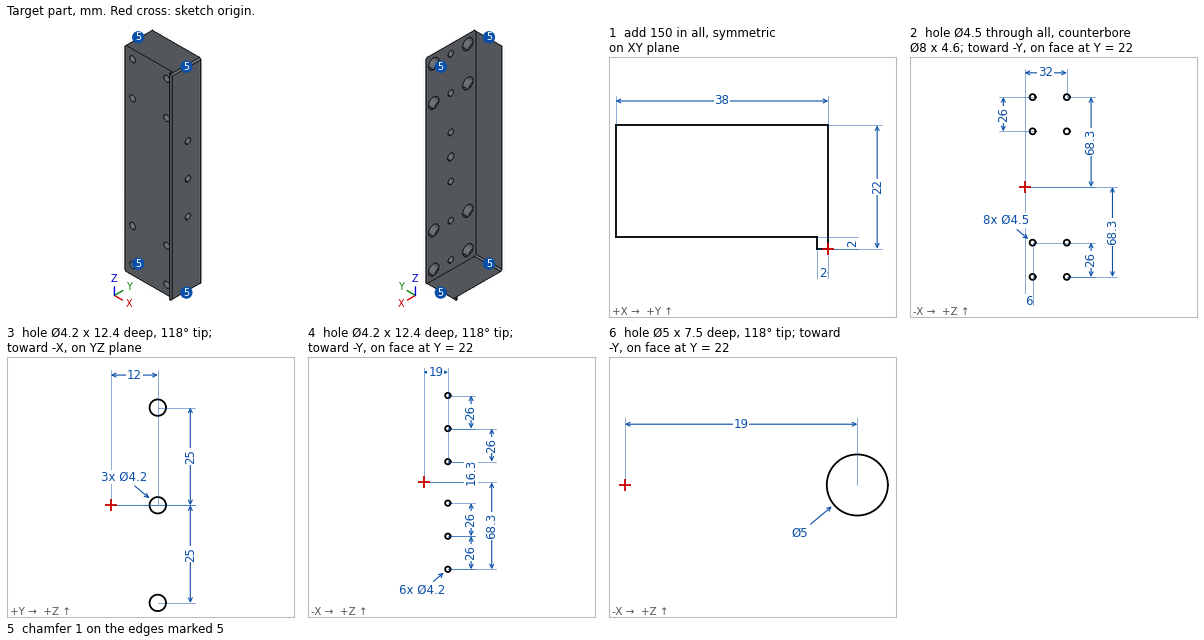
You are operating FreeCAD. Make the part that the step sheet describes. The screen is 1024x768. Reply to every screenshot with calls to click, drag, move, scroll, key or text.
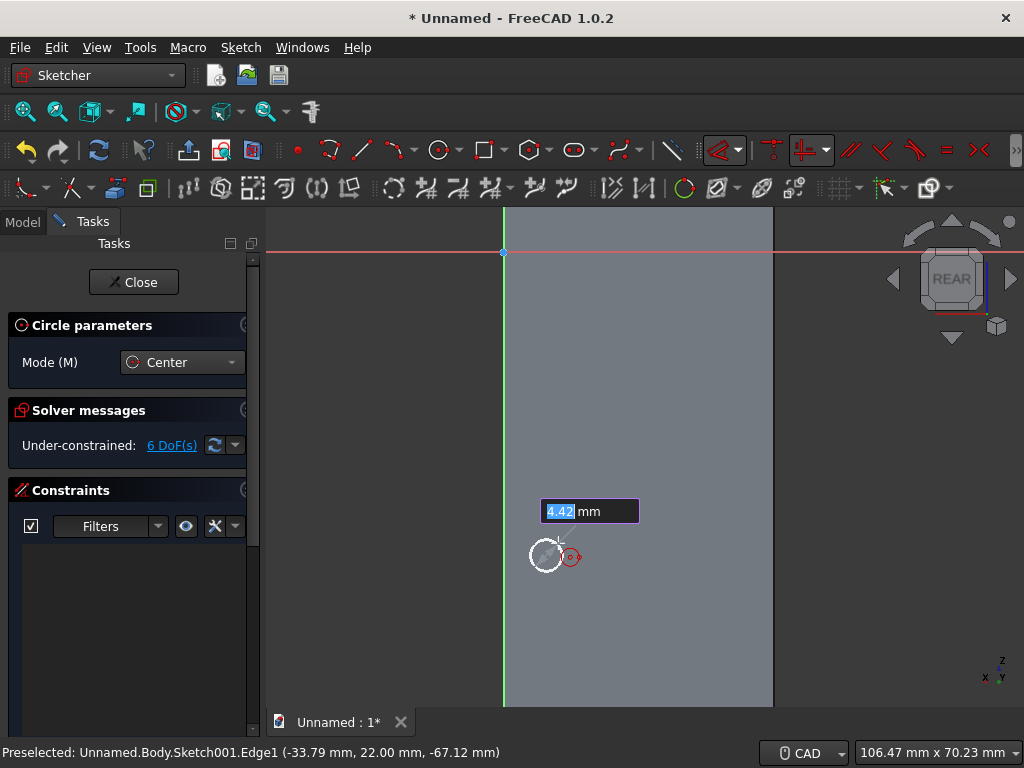
click(558, 542)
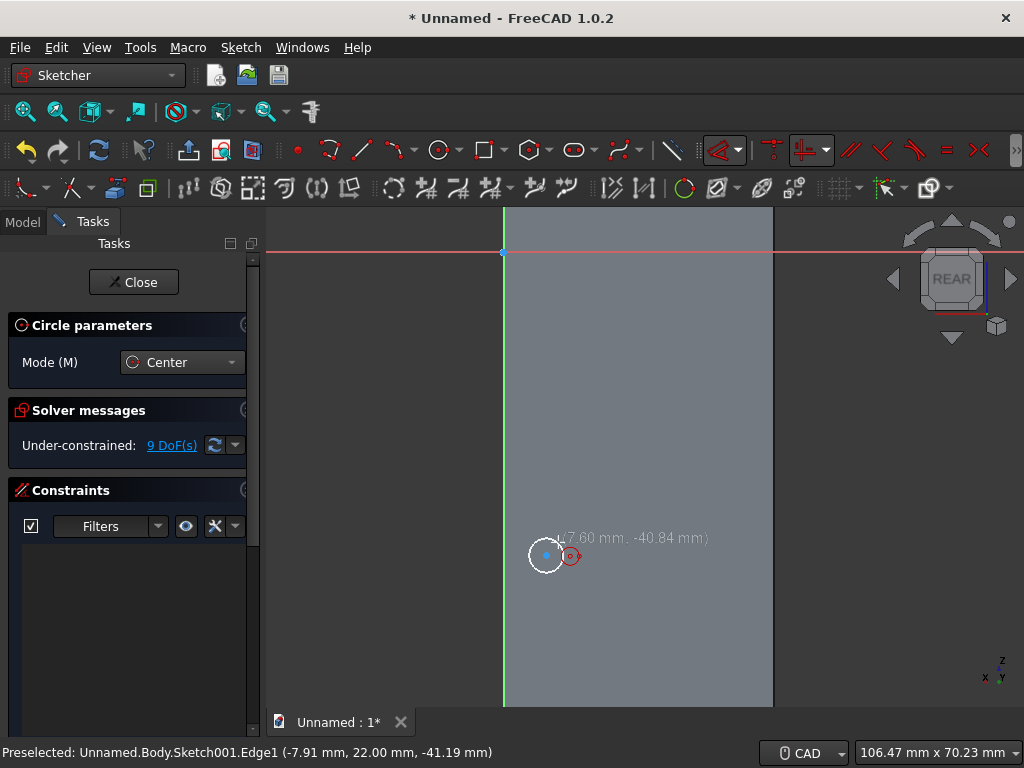
scroll(732, 553, up, 2)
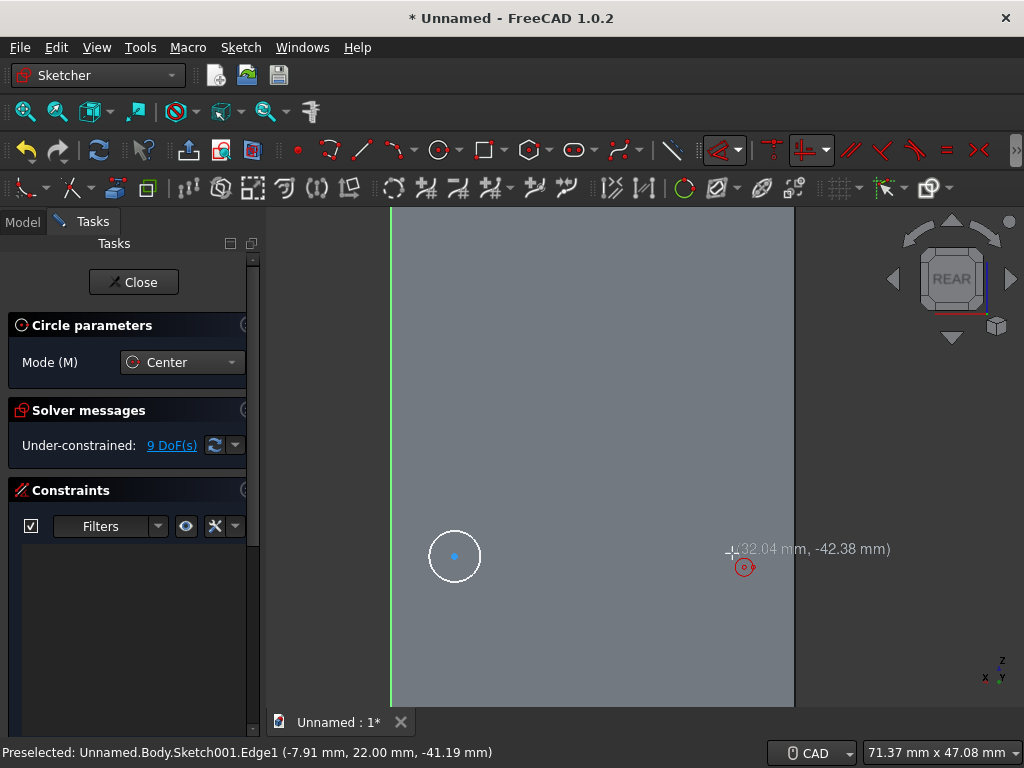
scroll(577, 546, down, 8)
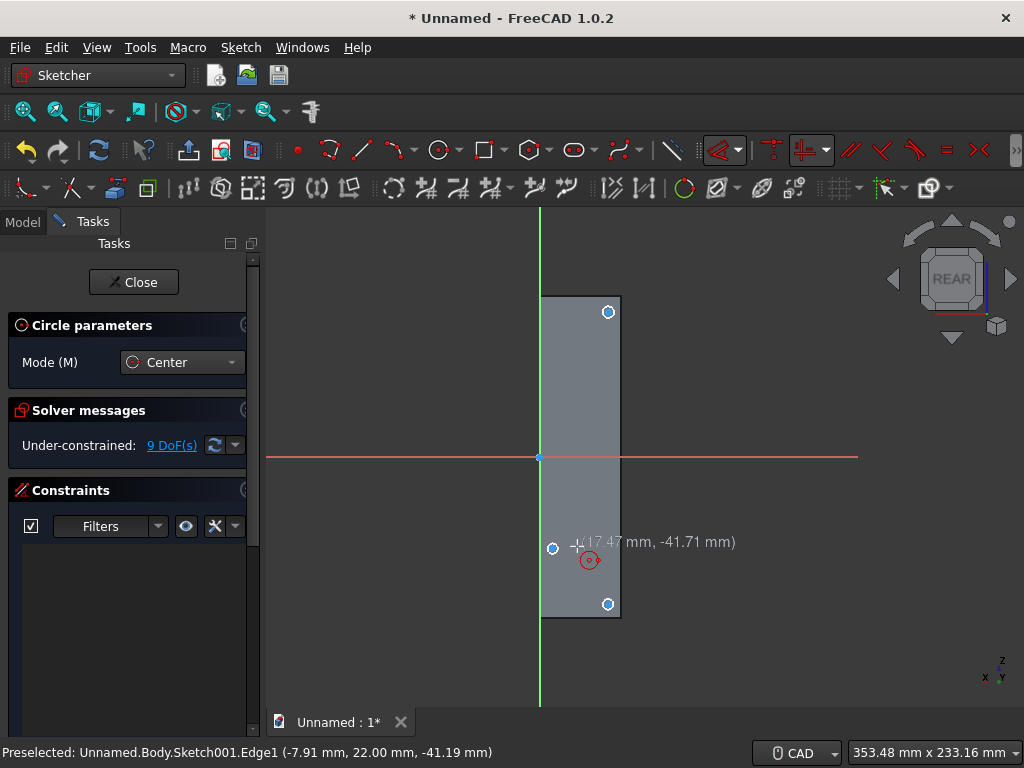
click(608, 548)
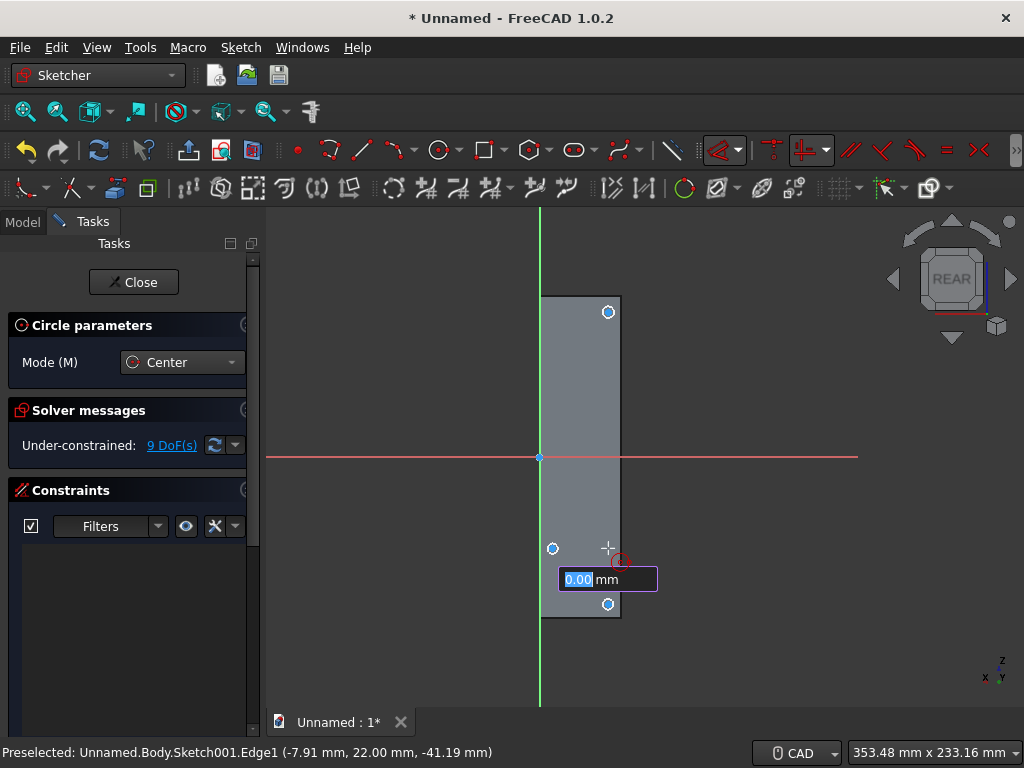
scroll(612, 545, up, 6)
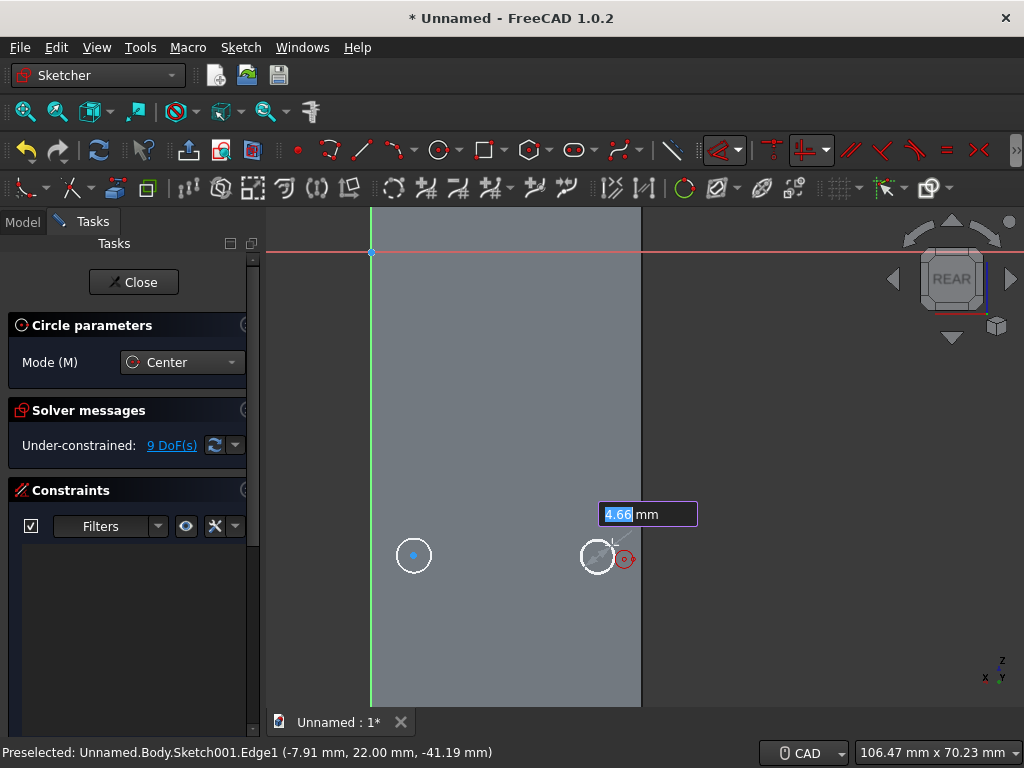
click(611, 542)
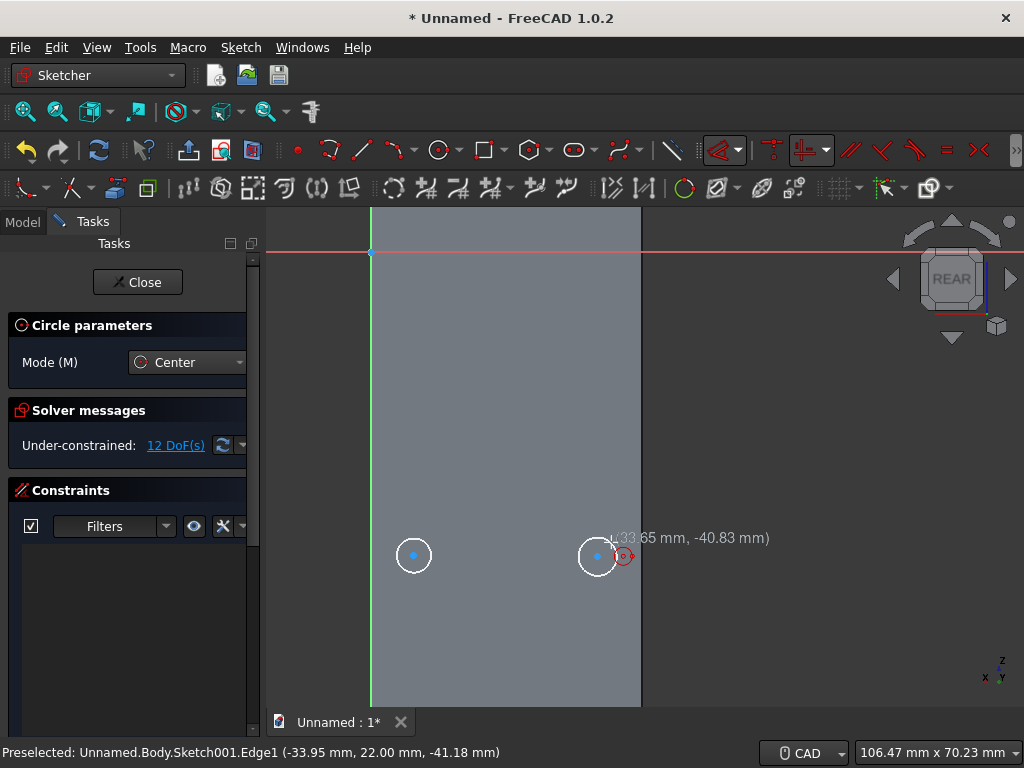
scroll(612, 545, down, 6)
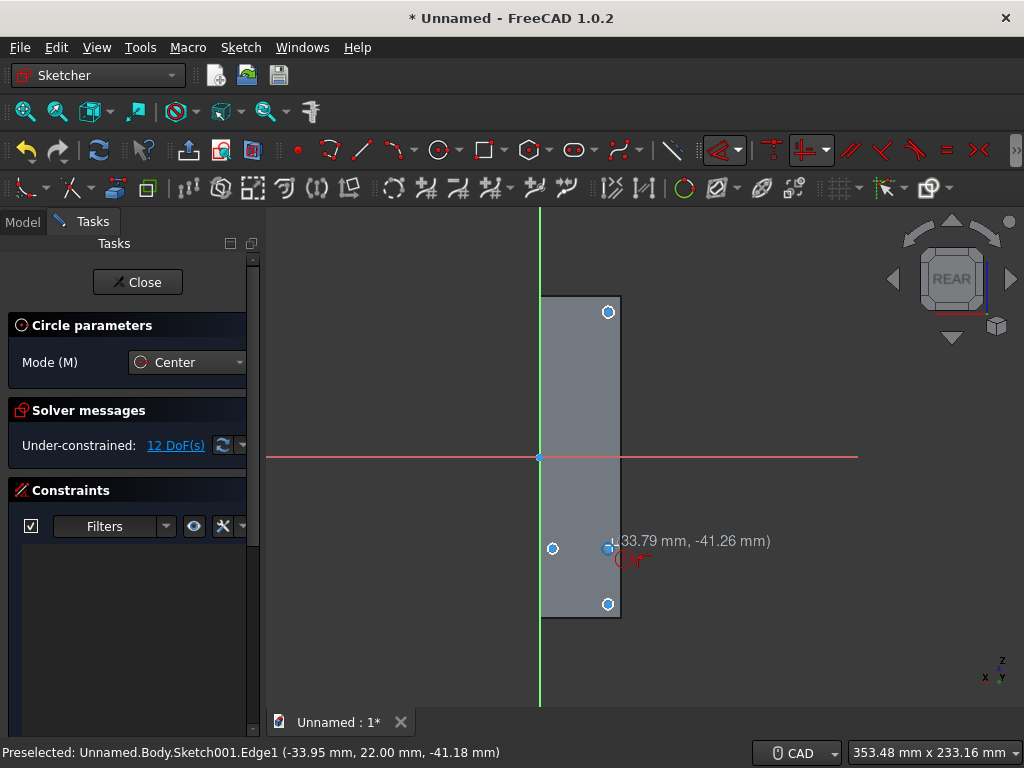
scroll(553, 604, up, 8)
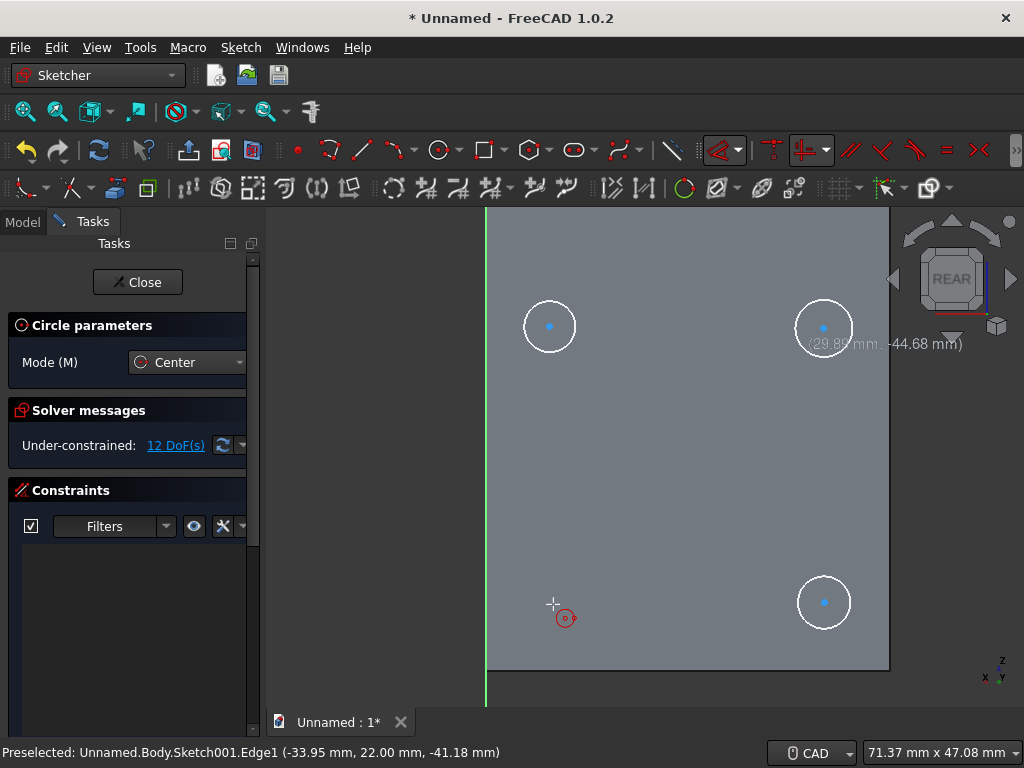
scroll(553, 604, down, 8)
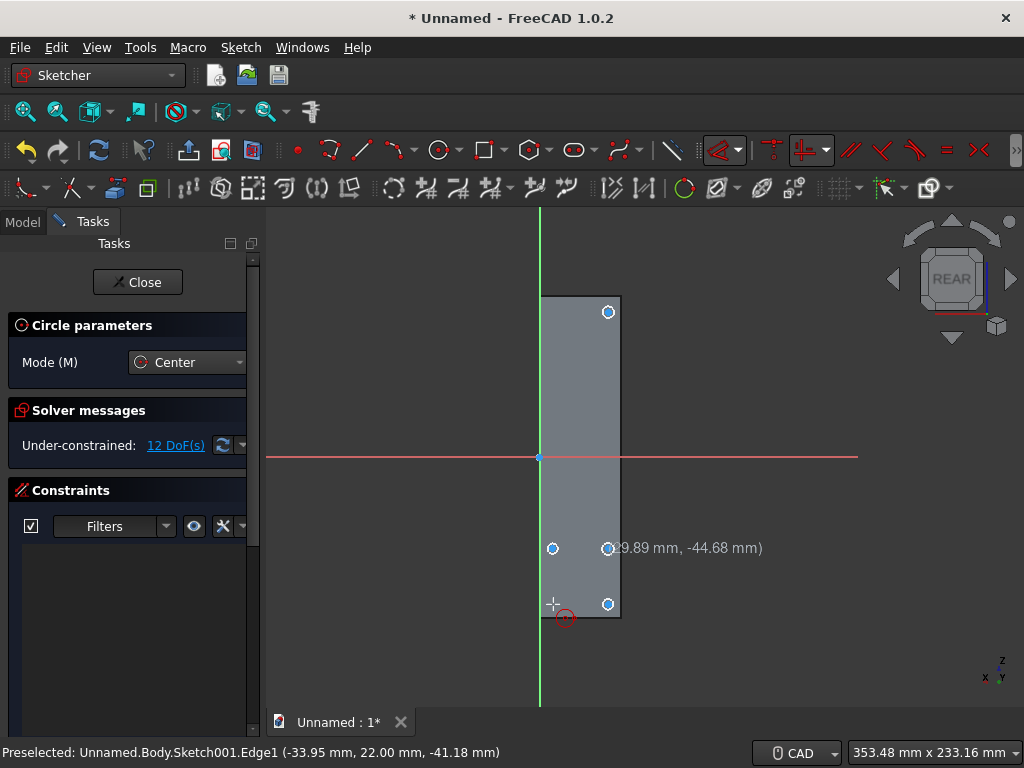
scroll(553, 604, up, 2)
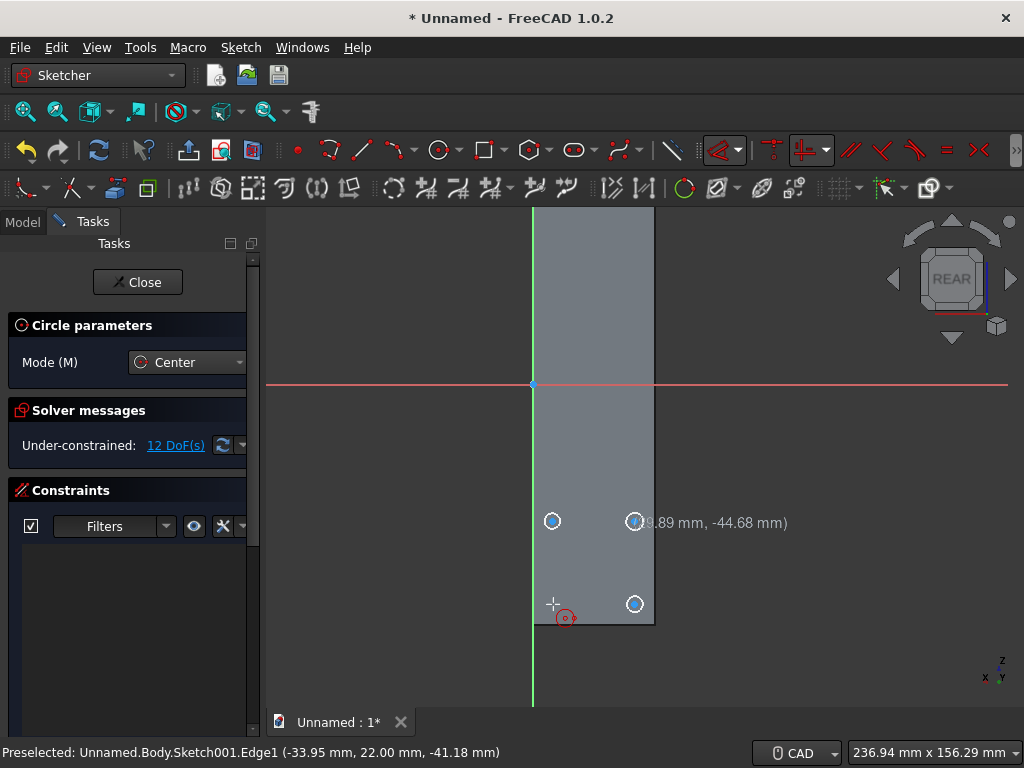
click(552, 603)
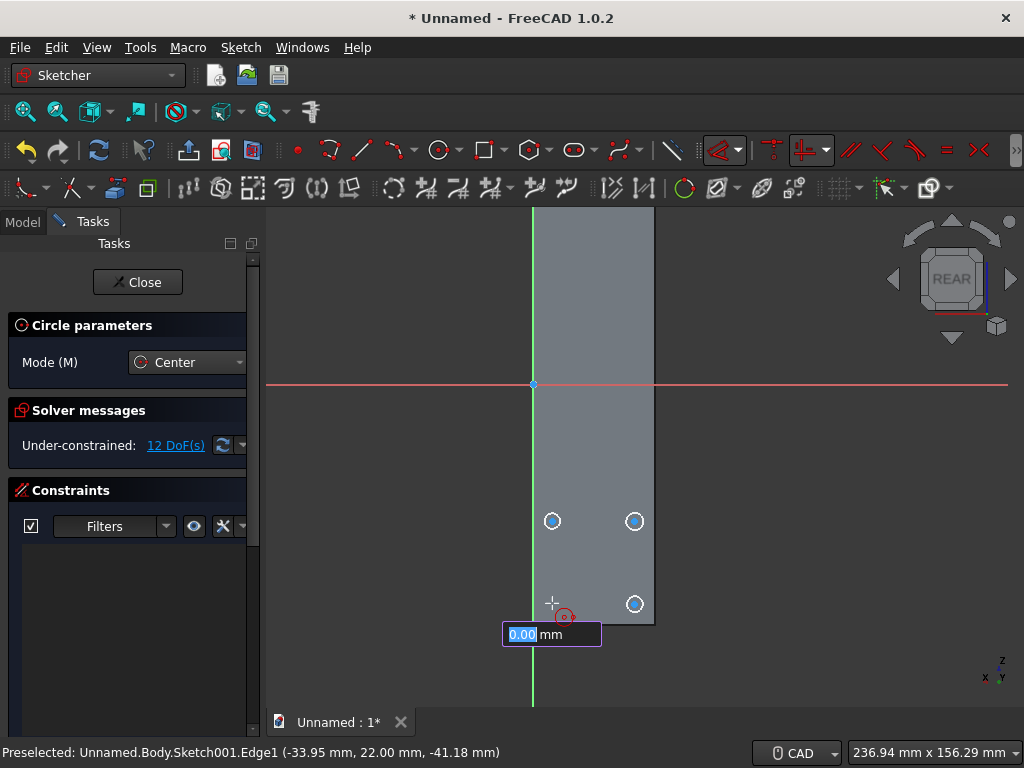
scroll(557, 598, up, 4)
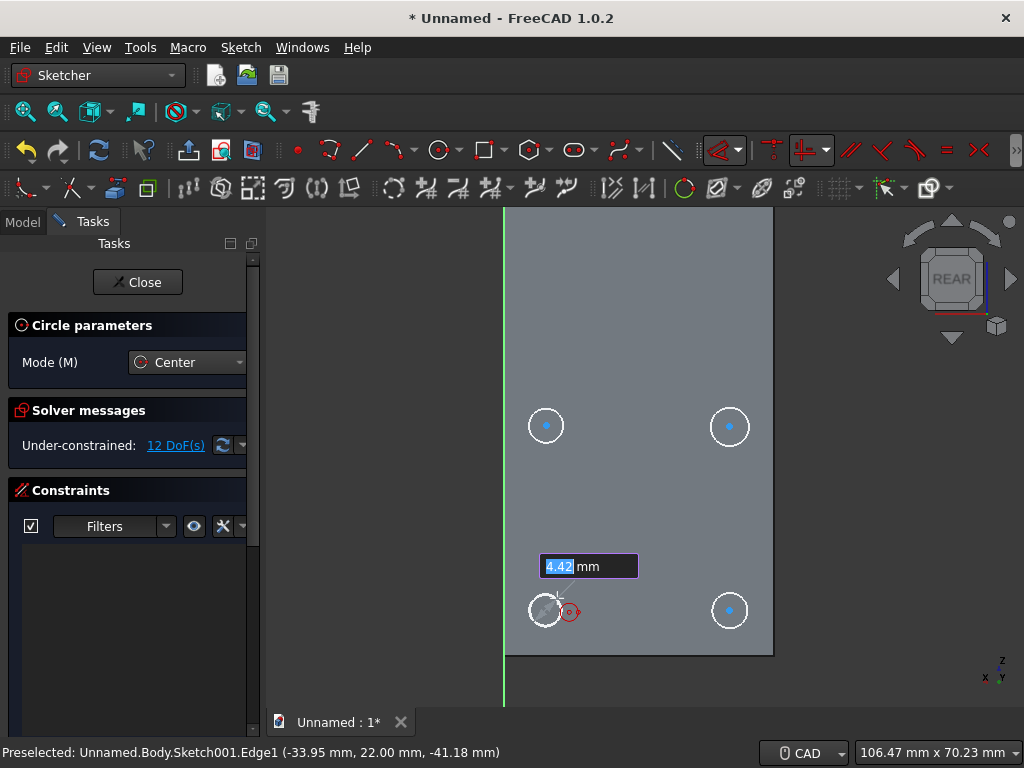
click(558, 597)